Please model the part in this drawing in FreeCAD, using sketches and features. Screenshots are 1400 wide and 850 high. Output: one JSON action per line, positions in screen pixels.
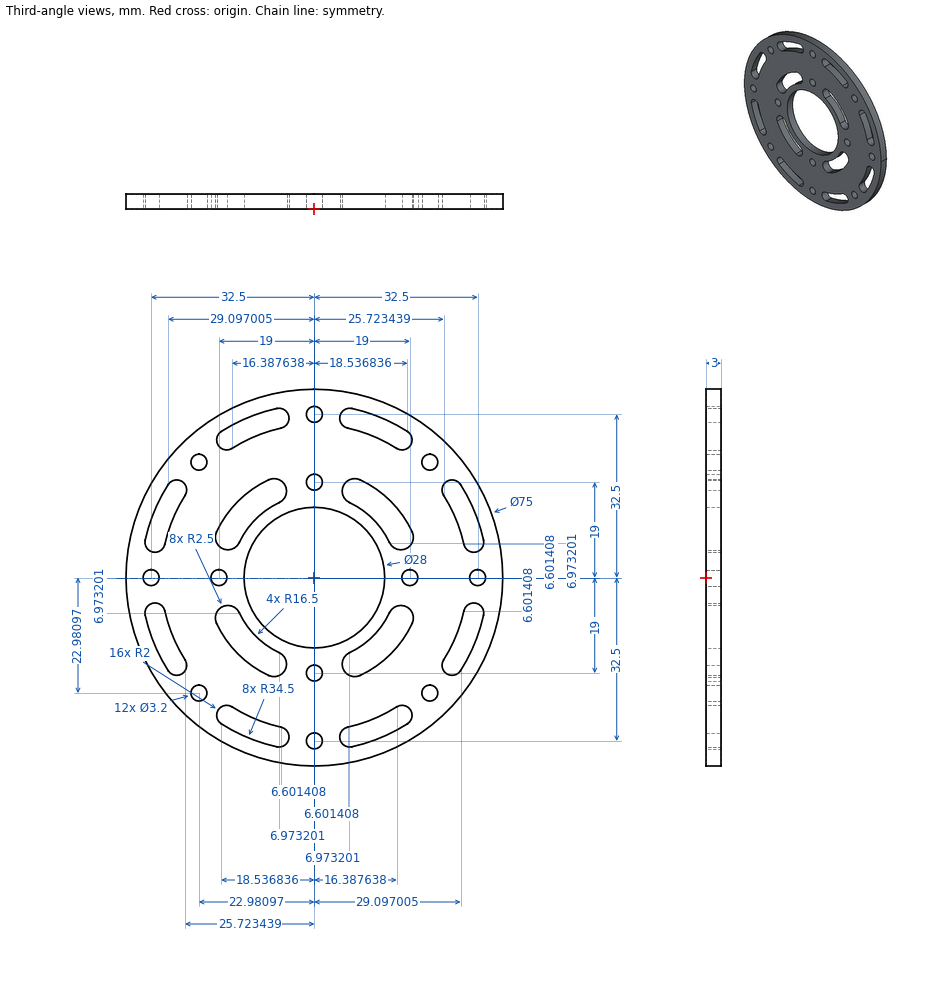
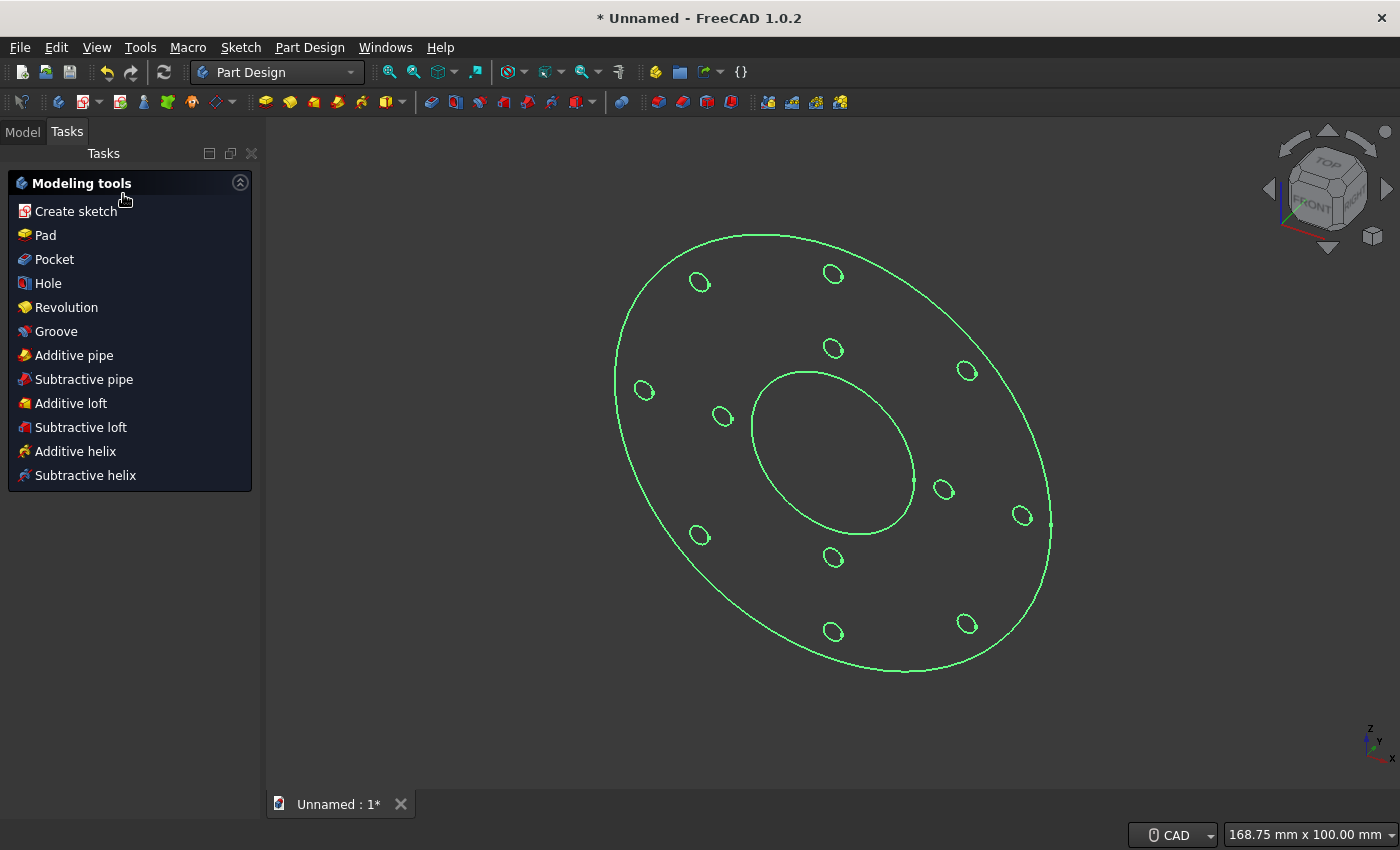
{"action": "left_click", "coordinate": [266, 102]}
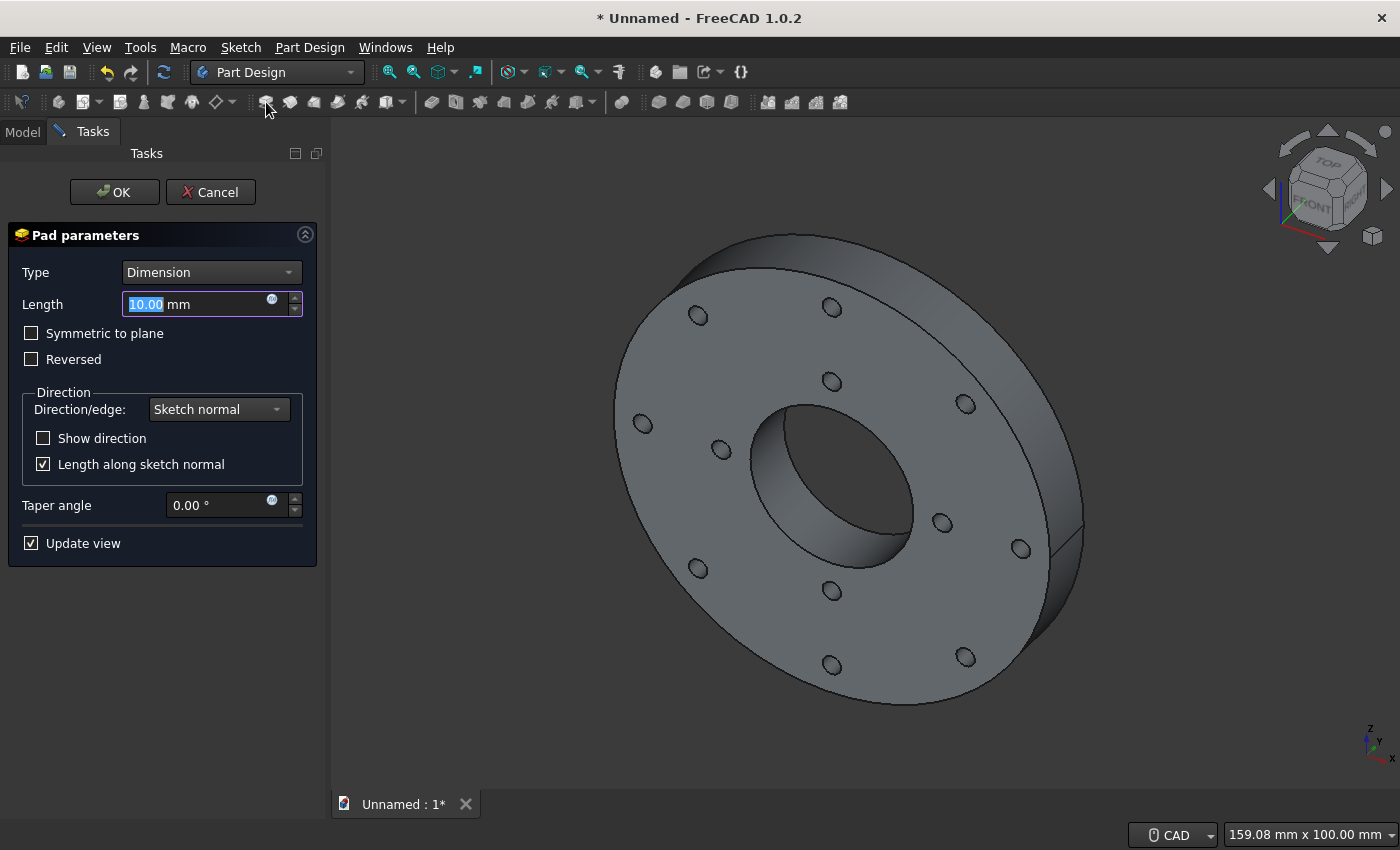
{"action": "type", "text": "3"}
{"action": "key", "text": "Tab"}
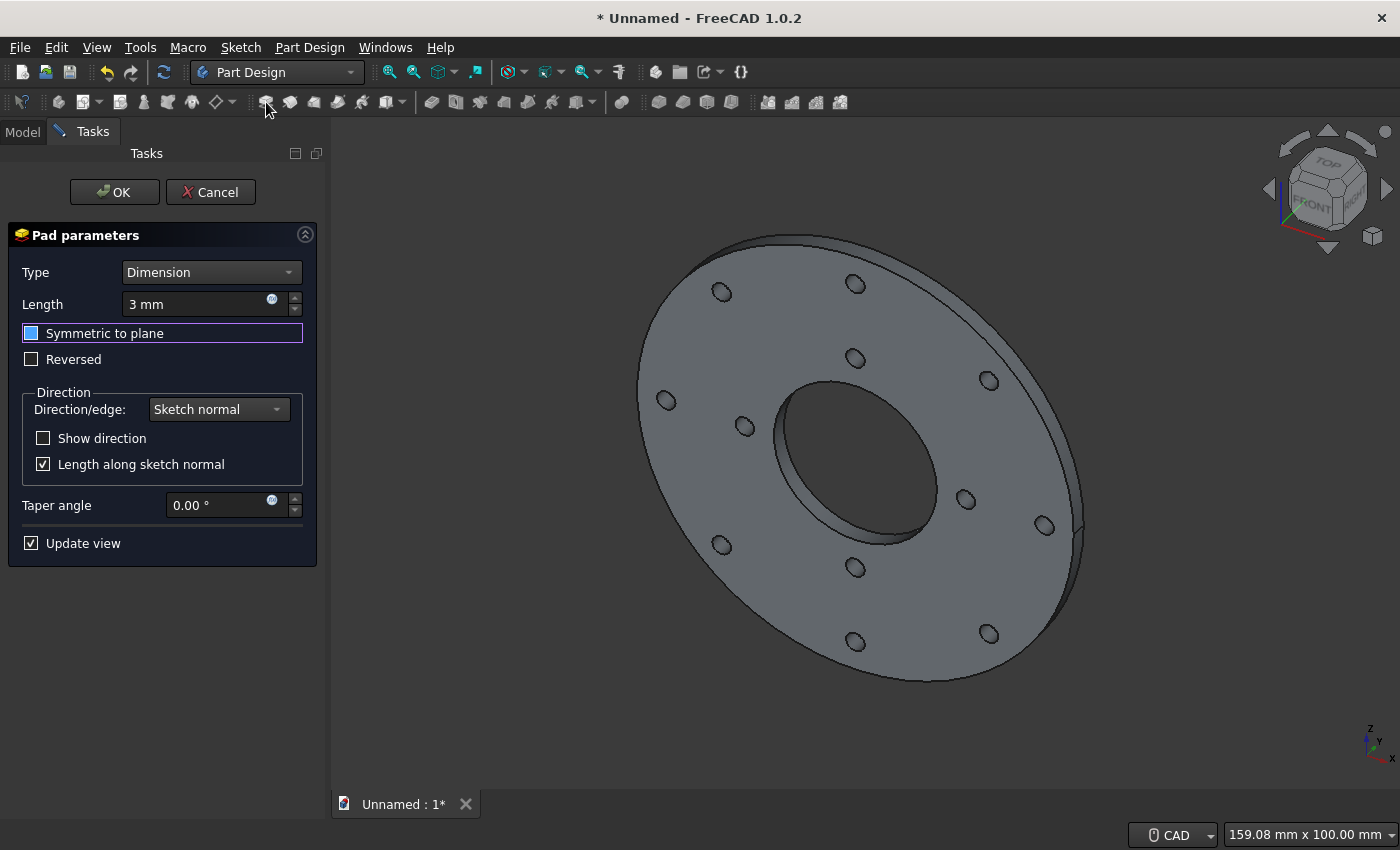
{"action": "left_click", "coordinate": [30, 359]}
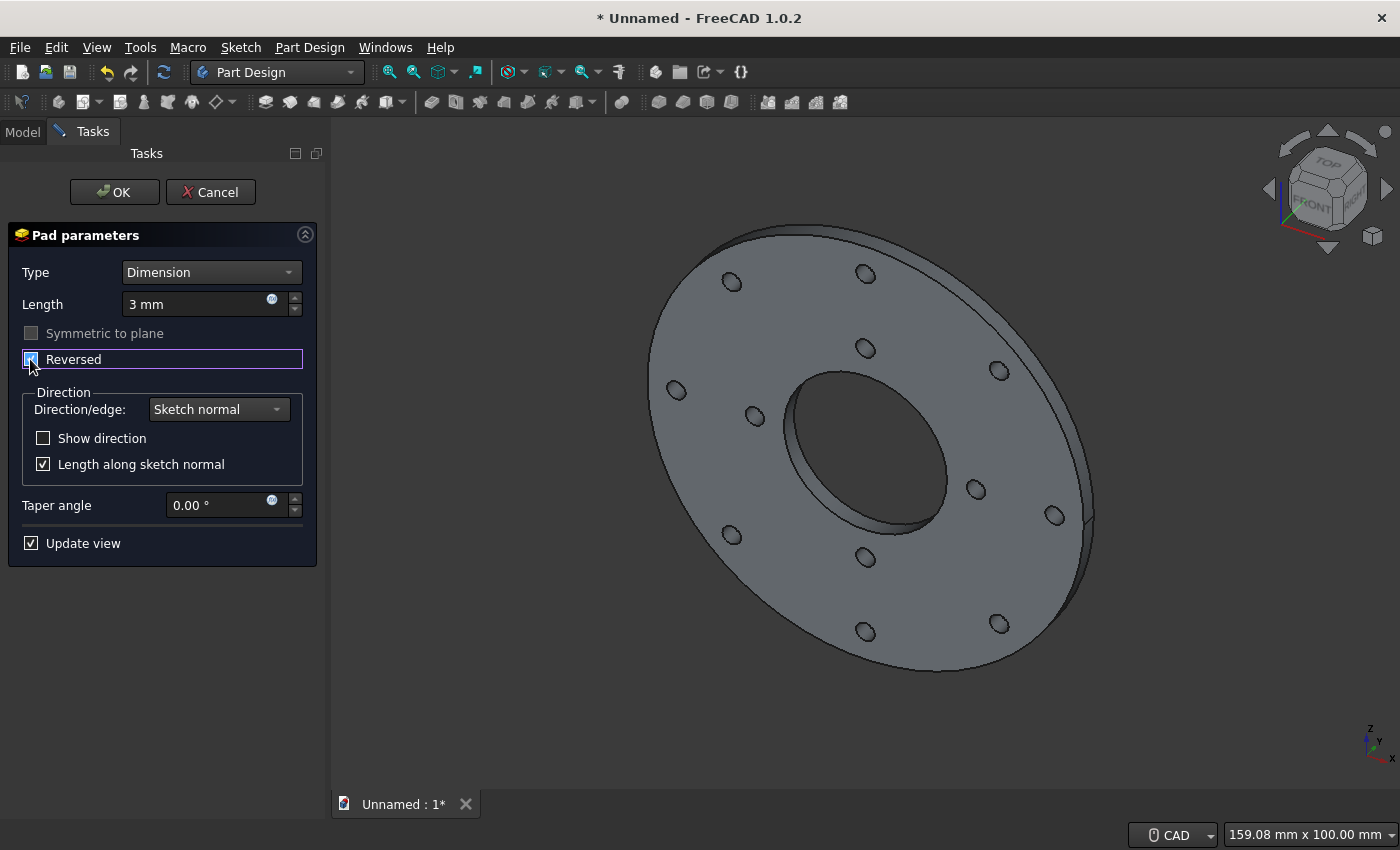
{"action": "left_click", "coordinate": [115, 192]}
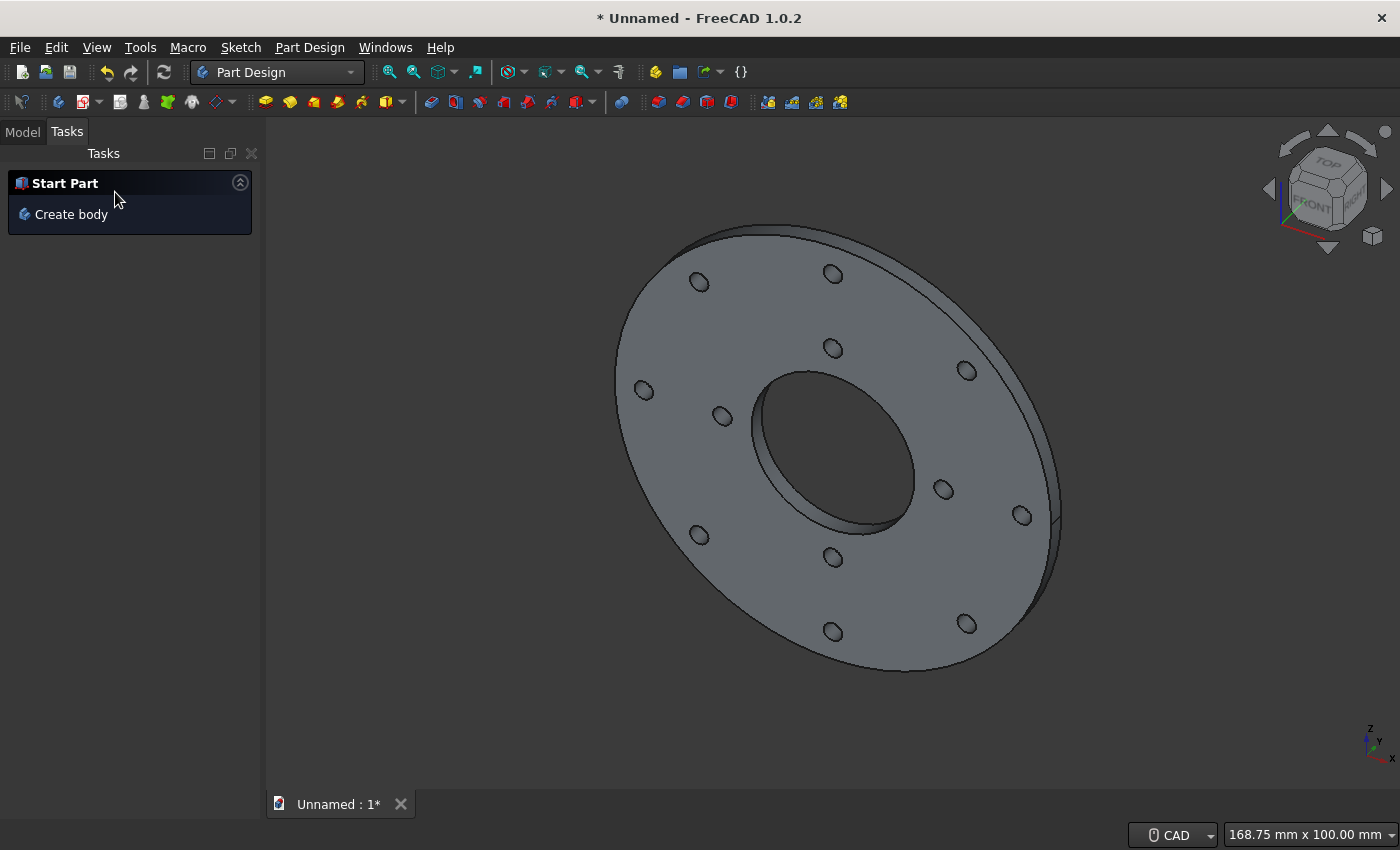
{"action": "key", "text": "4"}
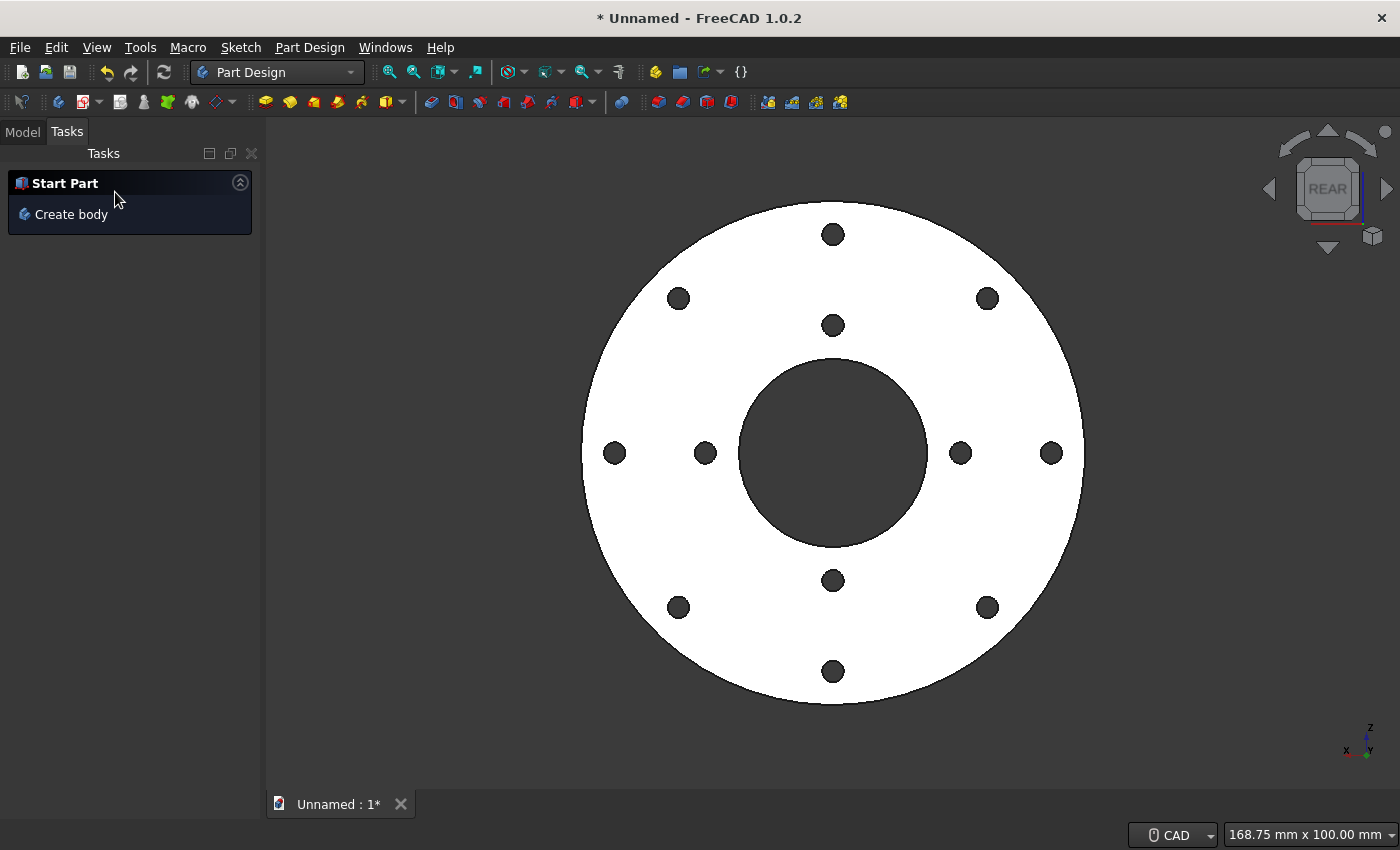
{"action": "left_click", "coordinate": [905, 308]}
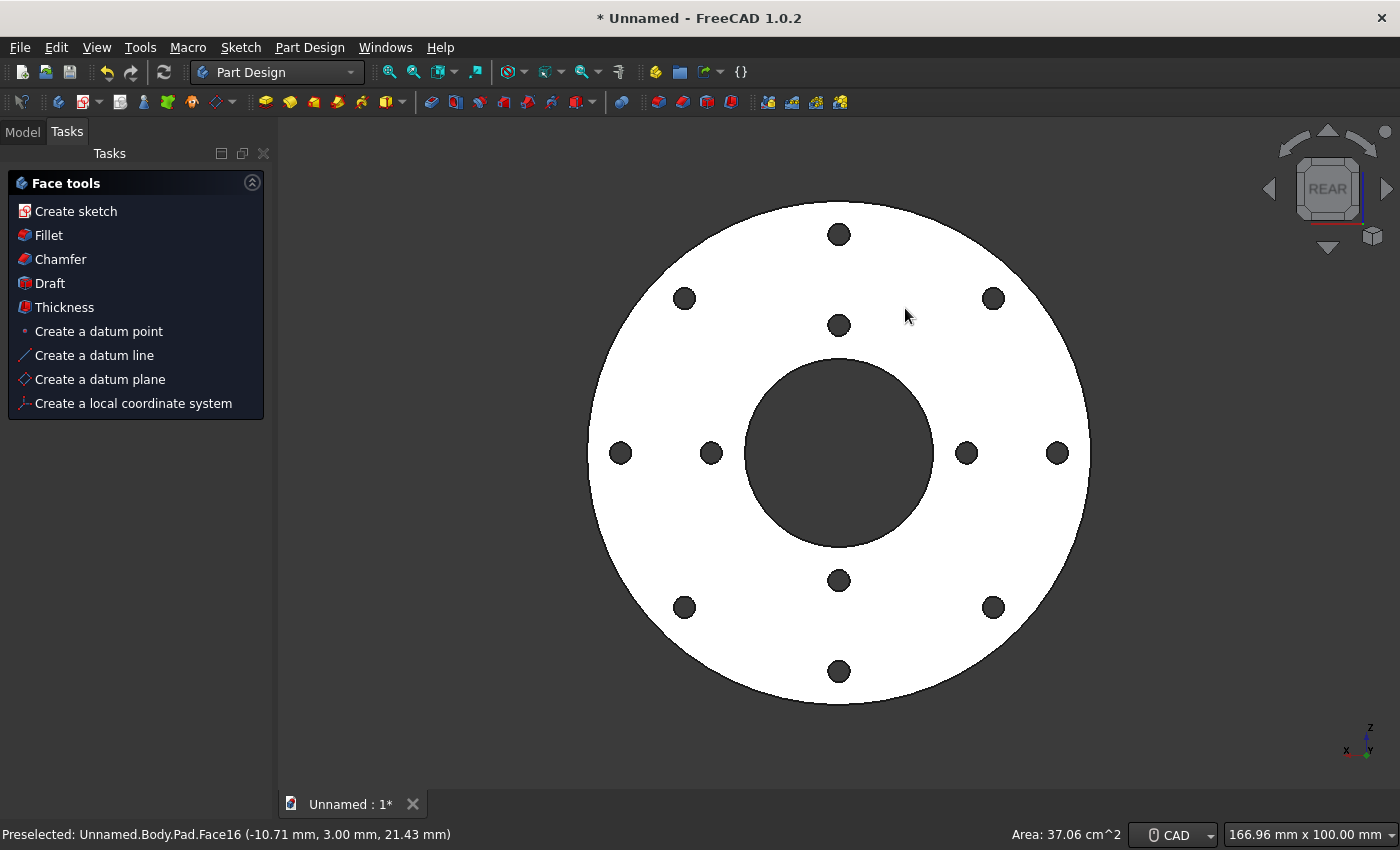
{"action": "left_click", "coordinate": [84, 102]}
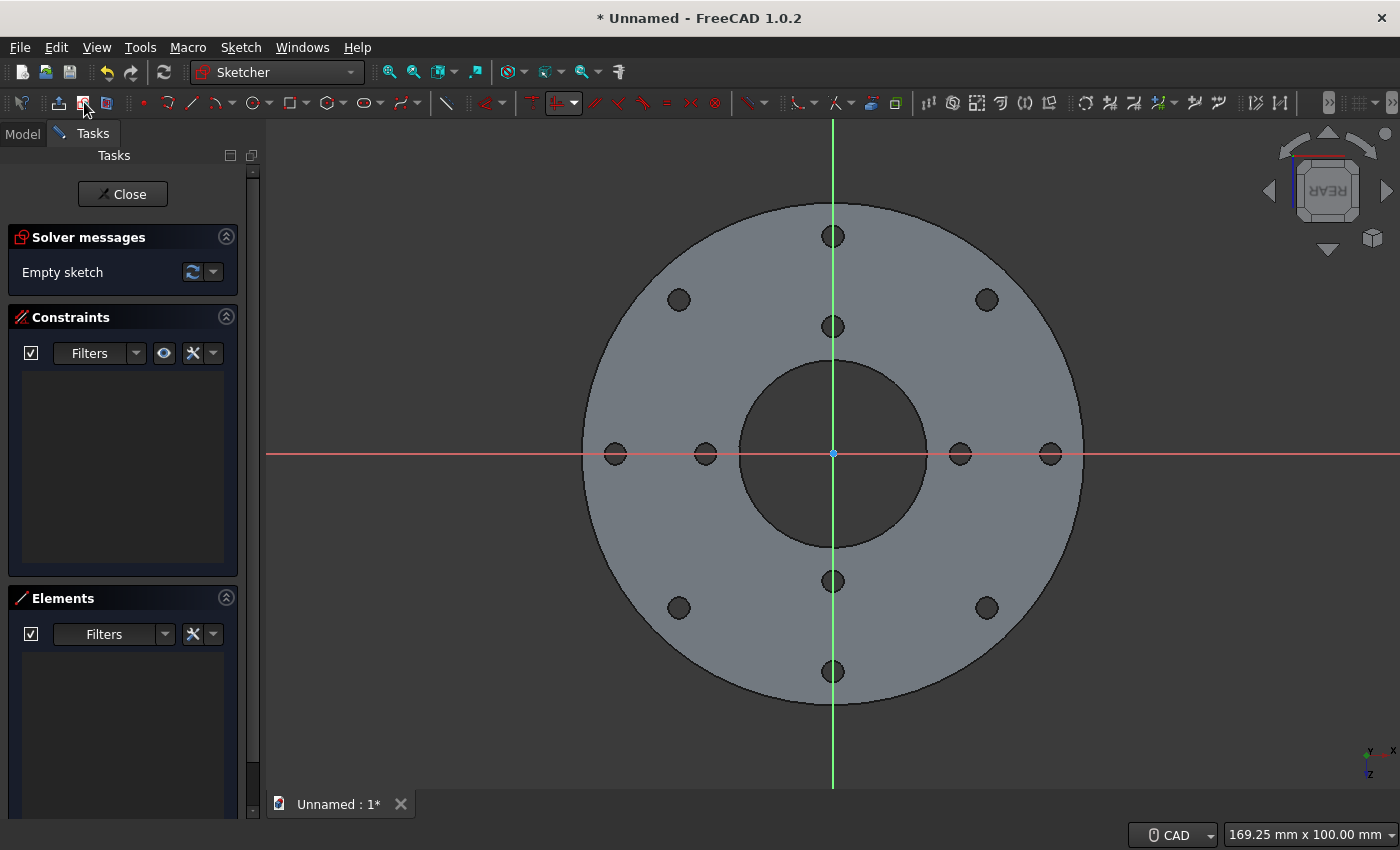
{"action": "key", "text": "g 3 a"}